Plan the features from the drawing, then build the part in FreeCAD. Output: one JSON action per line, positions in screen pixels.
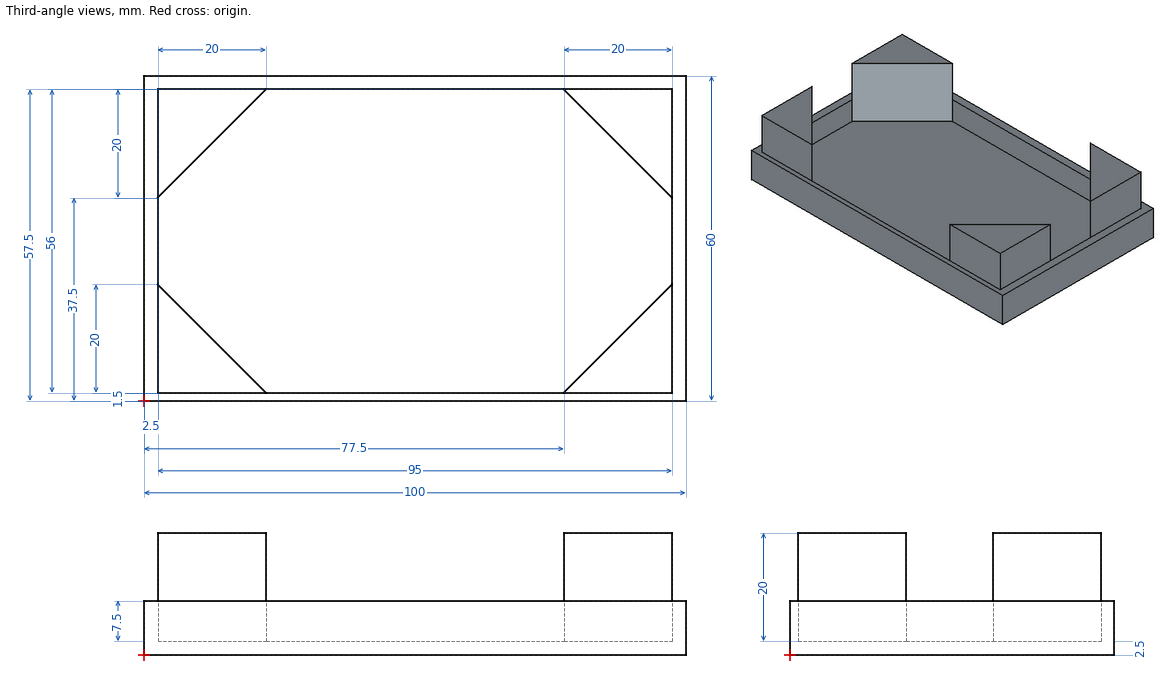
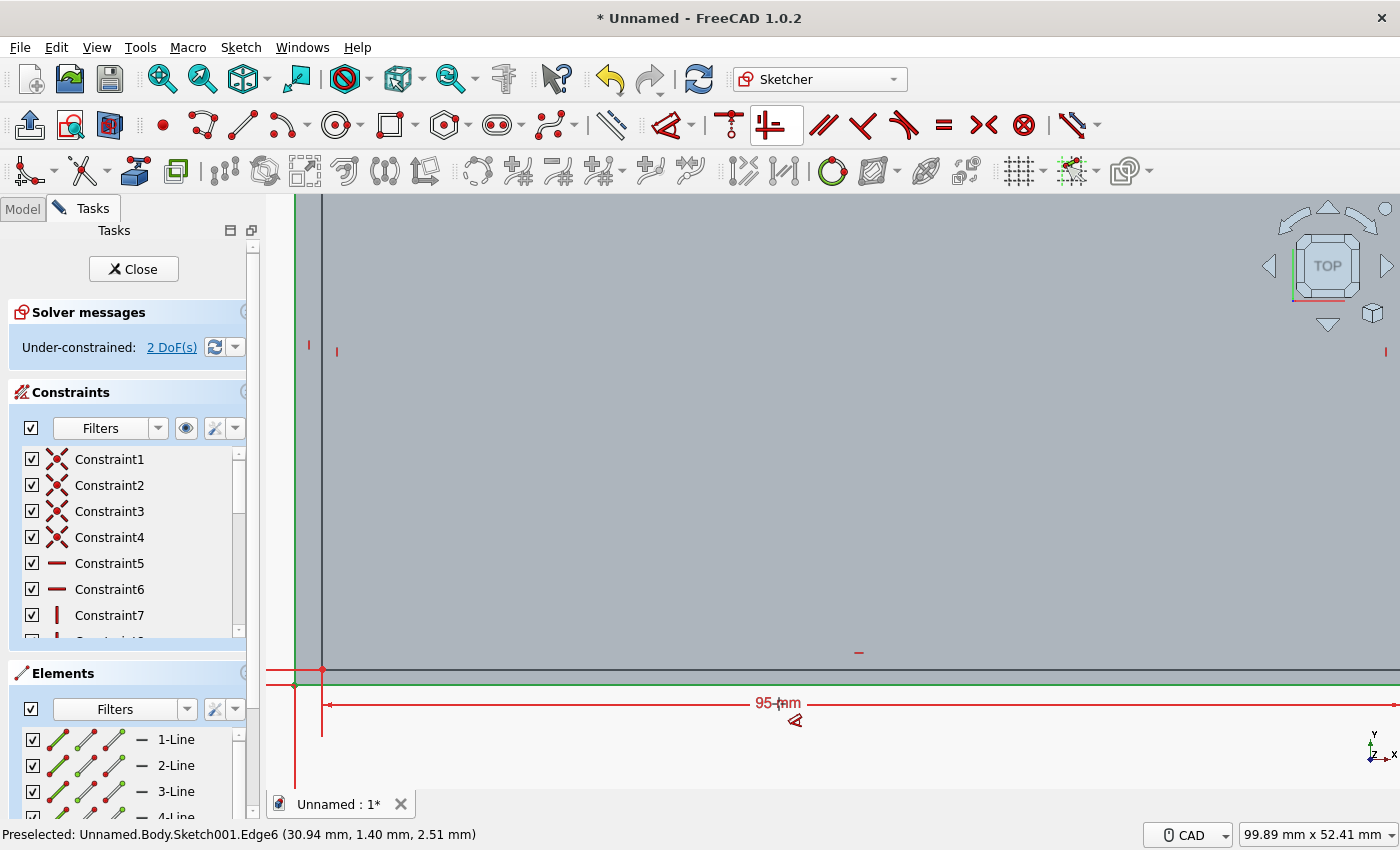
{"action": "scroll", "coordinate": [645, 670], "scroll_direction": "down", "scroll_amount": 3}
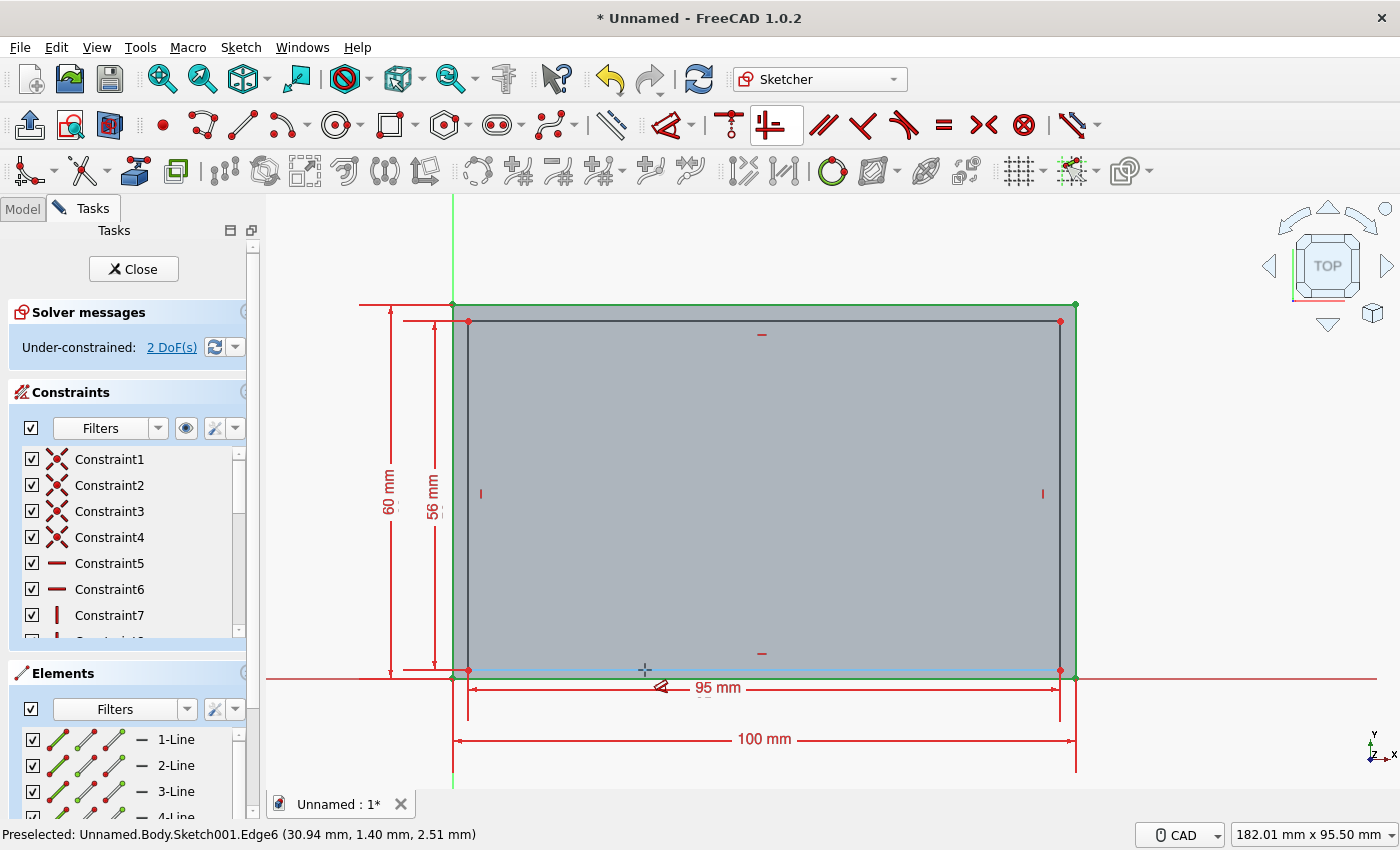
{"action": "scroll", "coordinate": [468, 321], "scroll_direction": "up", "scroll_amount": 5}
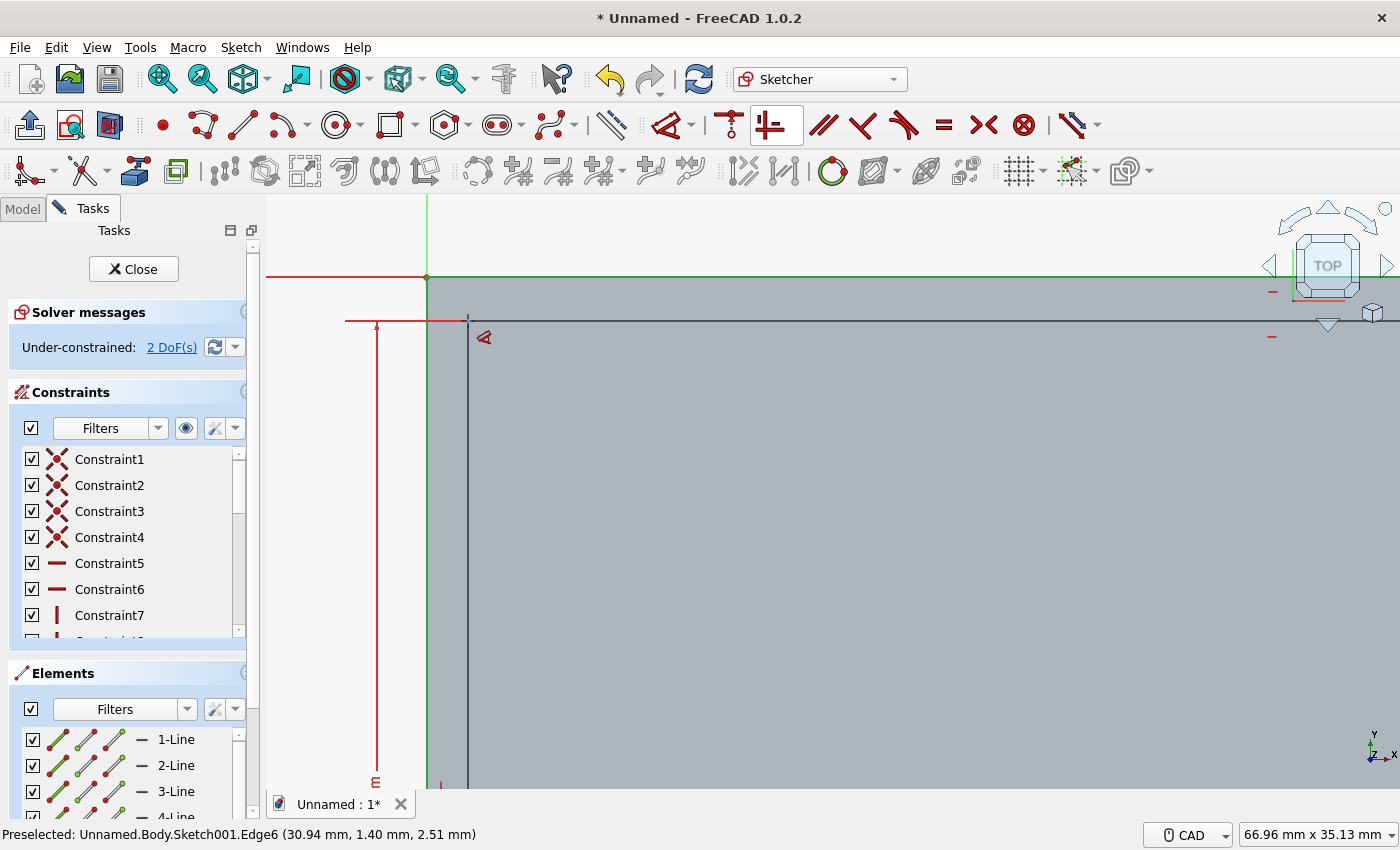
{"action": "left_click", "coordinate": [468, 321]}
{"action": "left_click", "coordinate": [447, 263]}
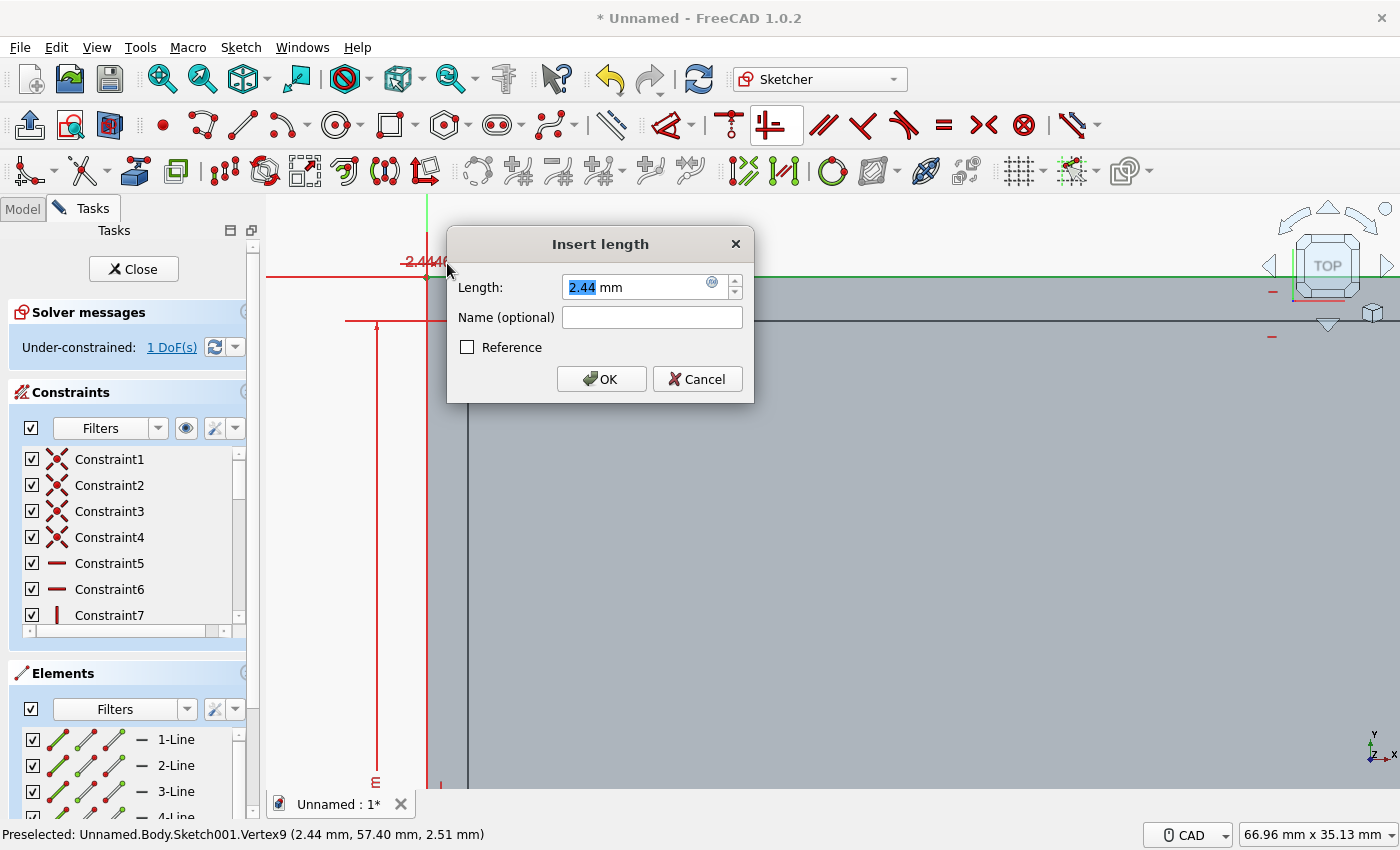
{"action": "type", "text": "2.5"}
{"action": "key", "text": "Return"}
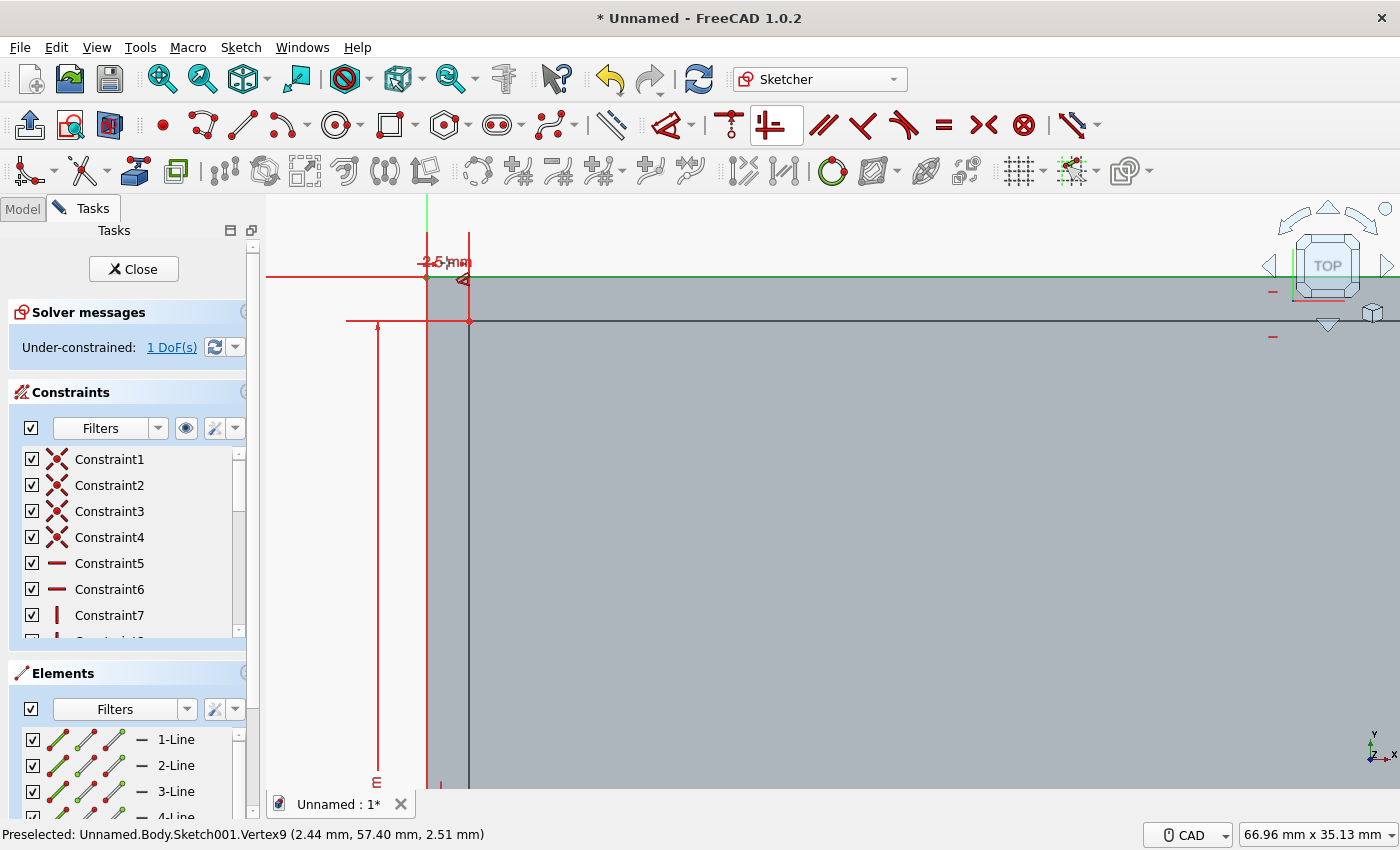
{"action": "scroll", "coordinate": [468, 321], "scroll_direction": "down", "scroll_amount": 5}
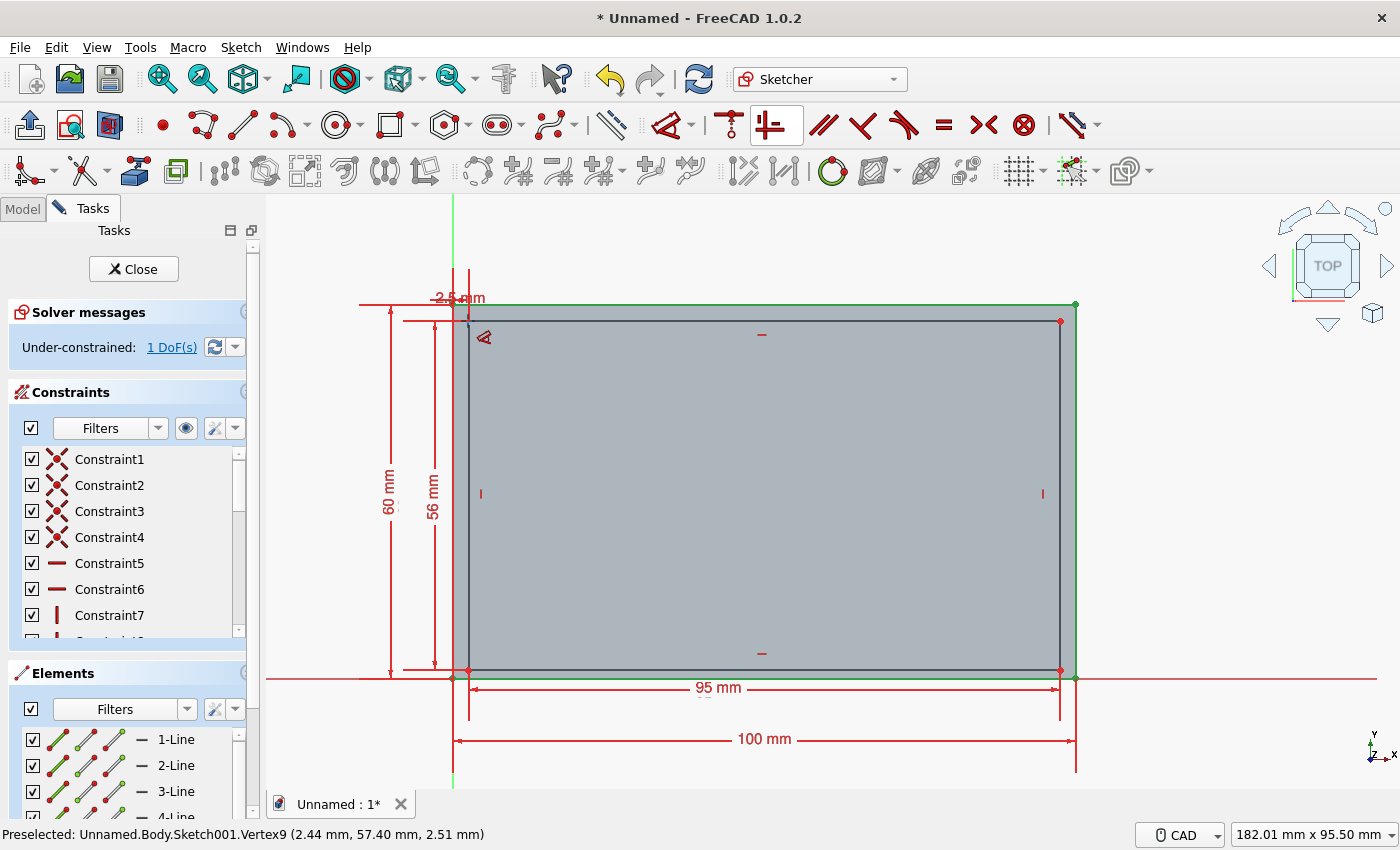
{"action": "scroll", "coordinate": [469, 670], "scroll_direction": "up", "scroll_amount": 8}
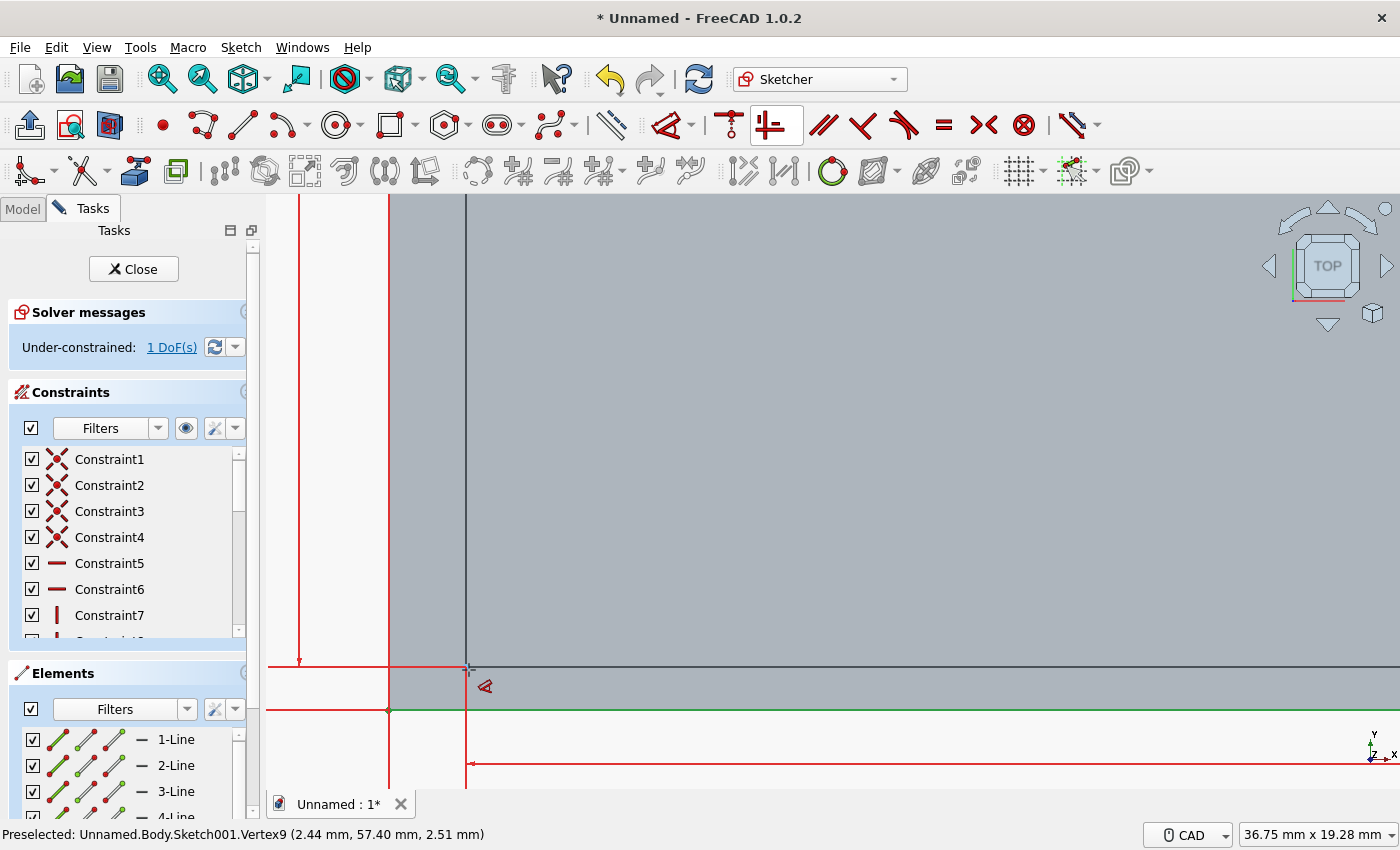
{"action": "left_click", "coordinate": [466, 667]}
{"action": "left_click", "coordinate": [355, 689]}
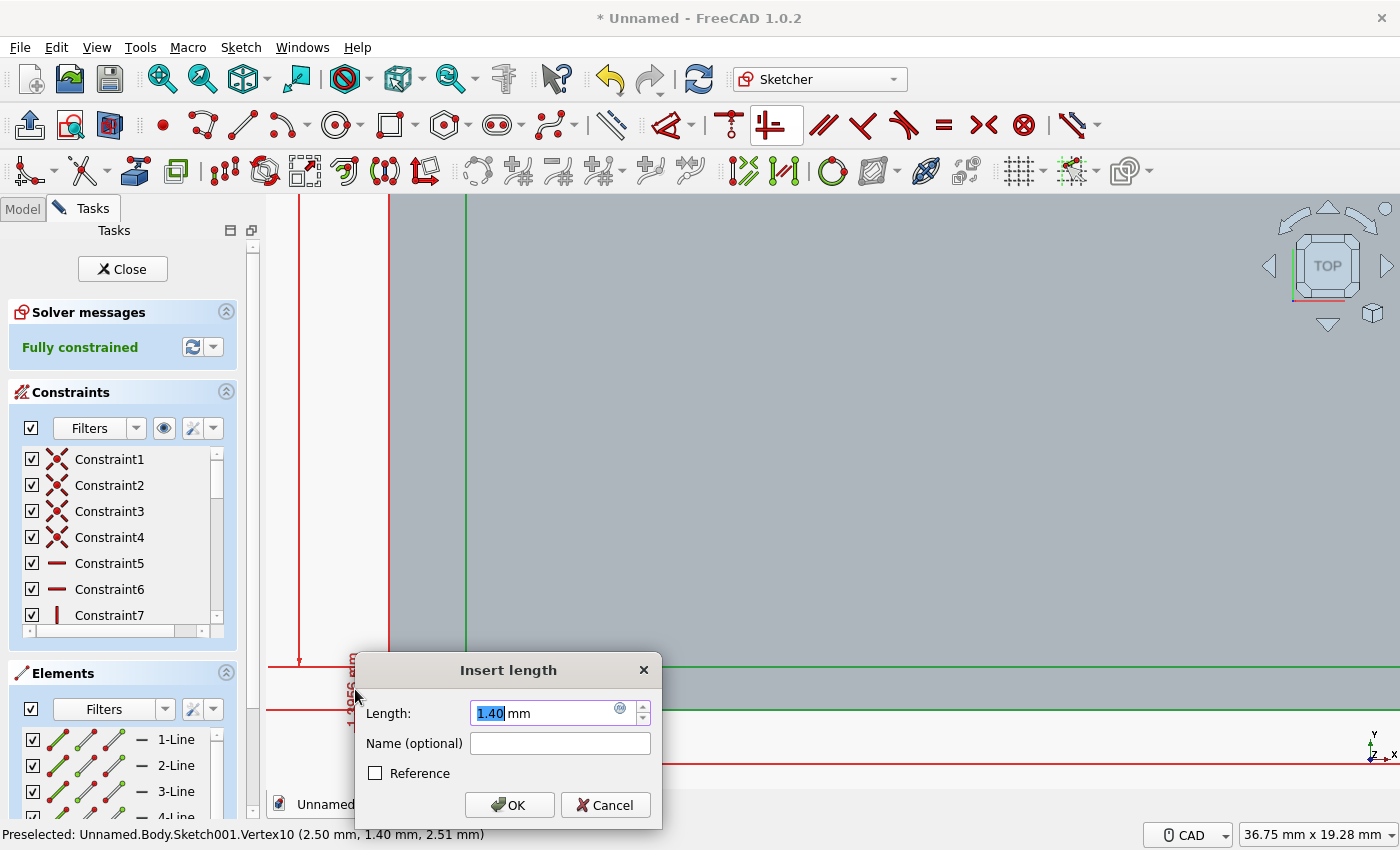
{"action": "type", "text": "1.5"}
{"action": "key", "text": "Return"}
{"action": "key", "text": "Escape"}